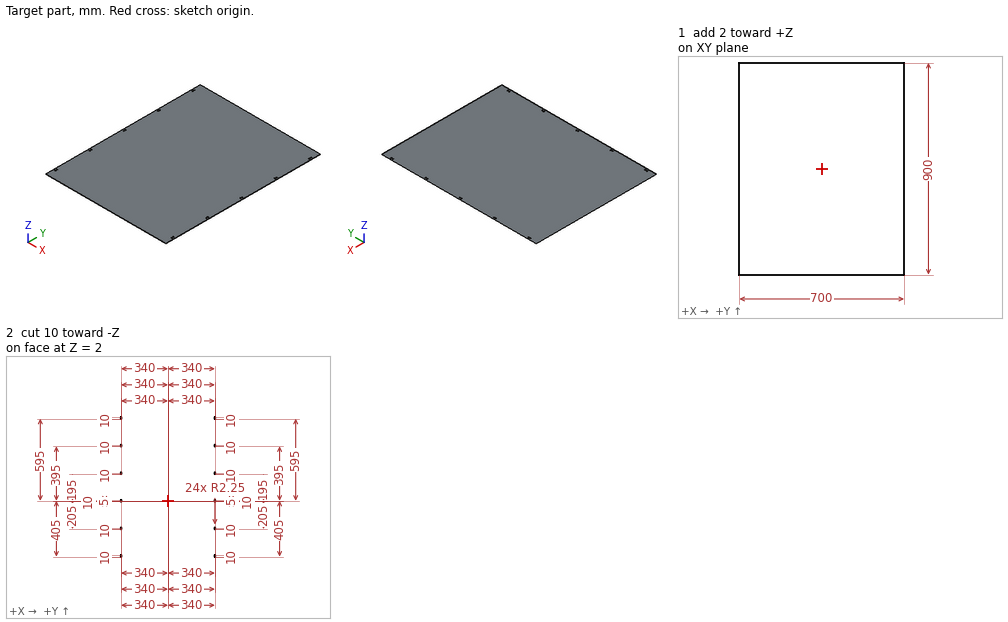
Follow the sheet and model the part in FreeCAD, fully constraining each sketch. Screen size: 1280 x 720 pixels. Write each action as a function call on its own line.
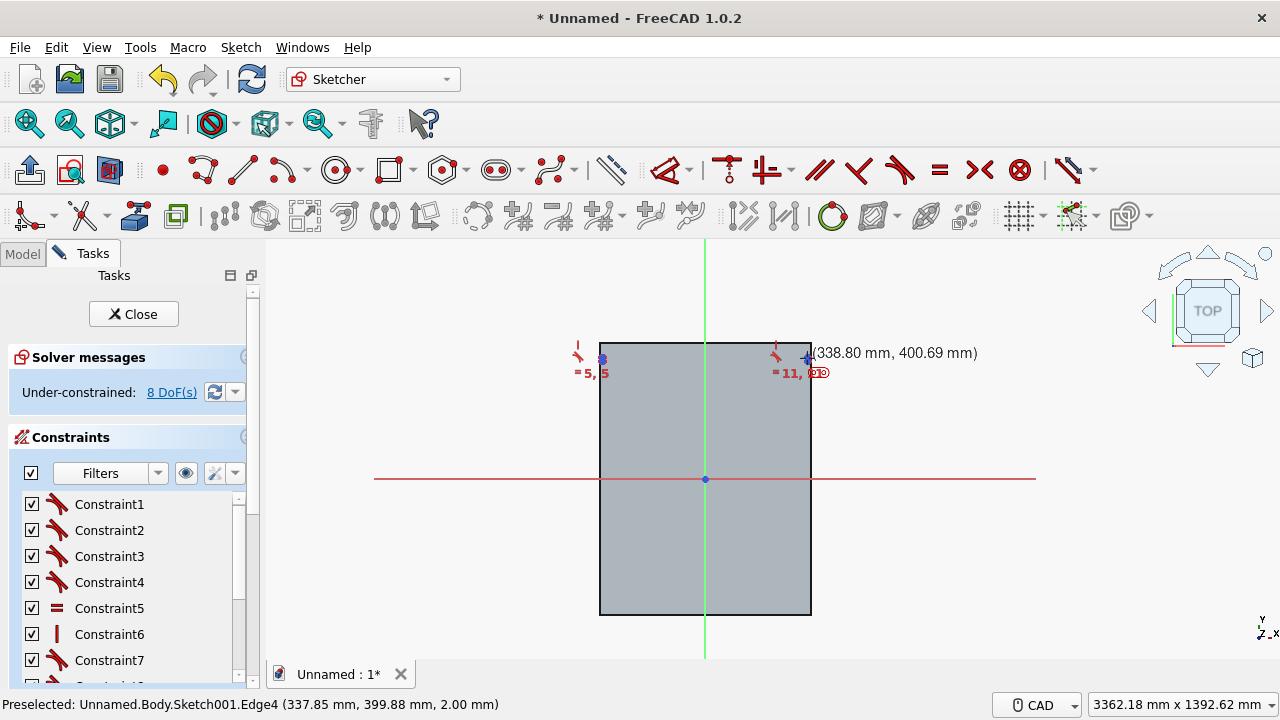
scroll(603, 420, up, 18)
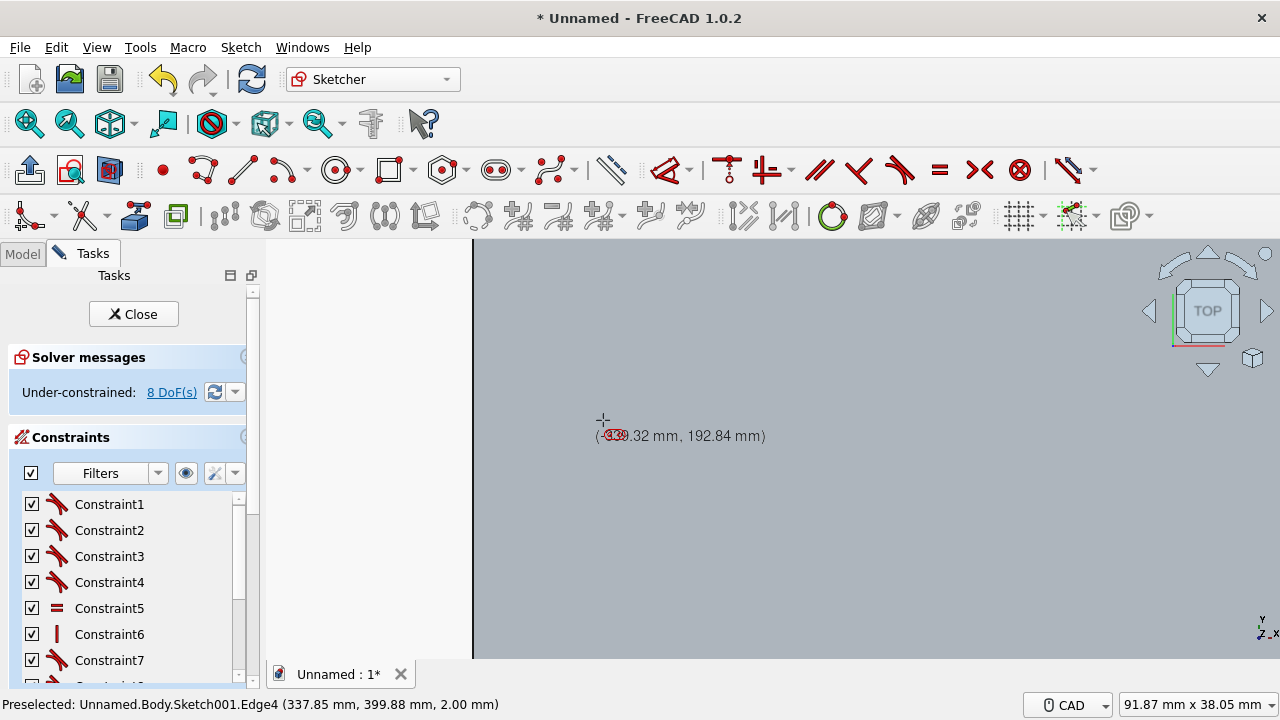
scroll(602, 420, down, 18)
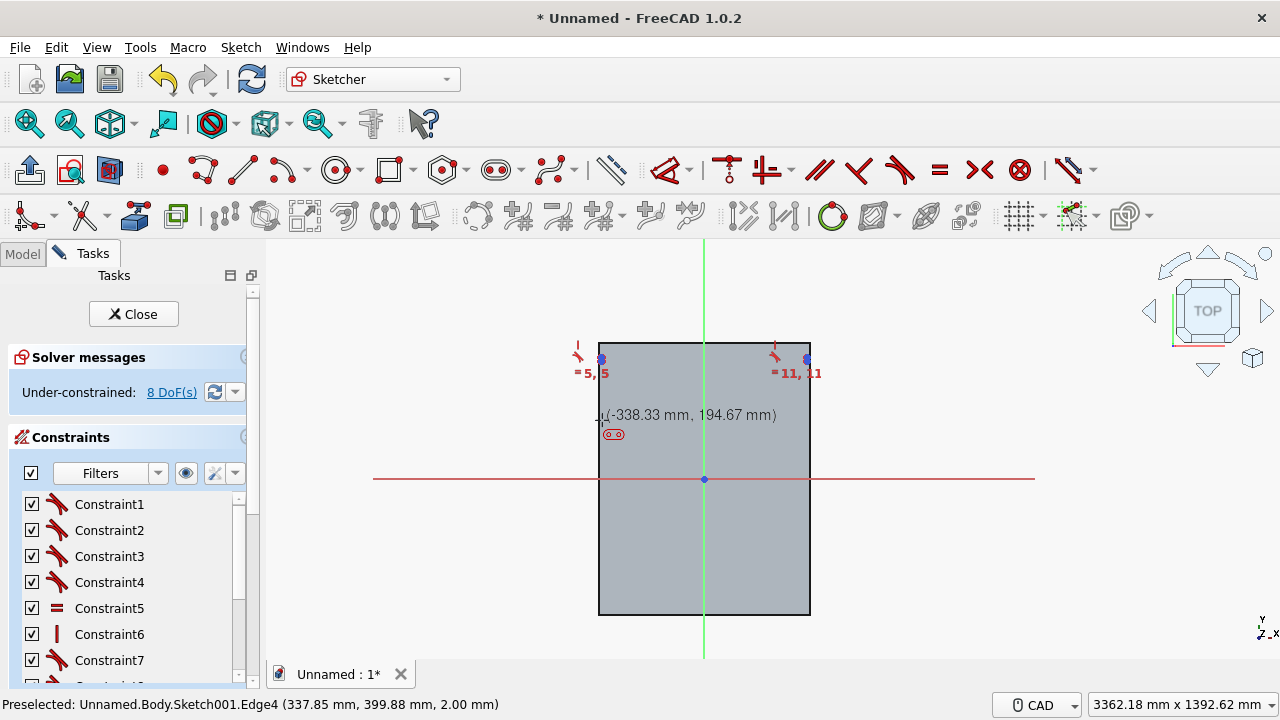
click(602, 420)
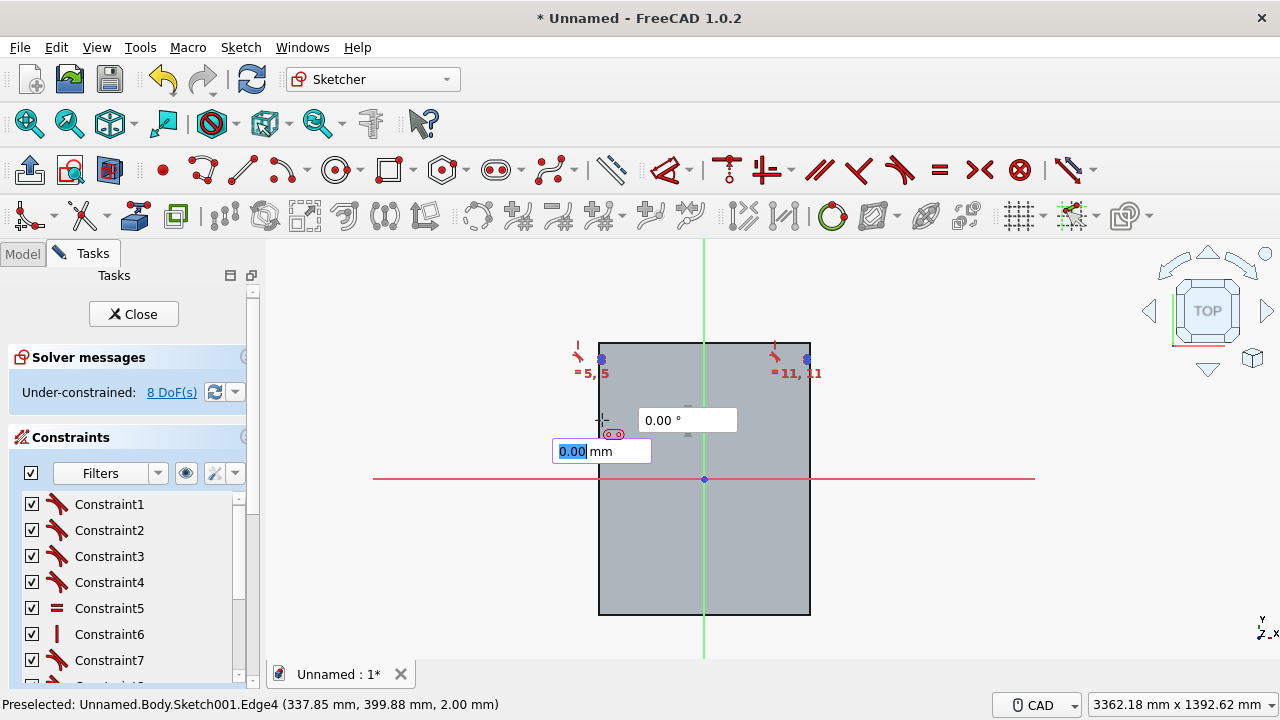
scroll(602, 417, up, 9)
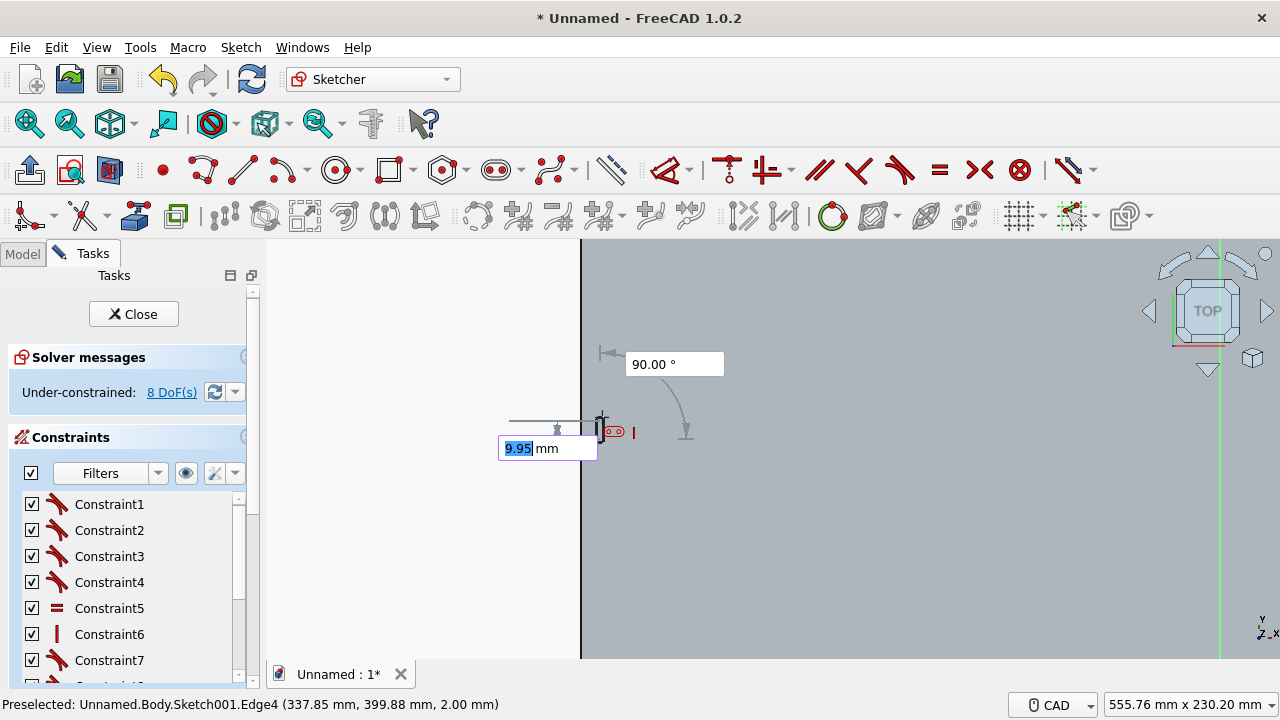
click(600, 417)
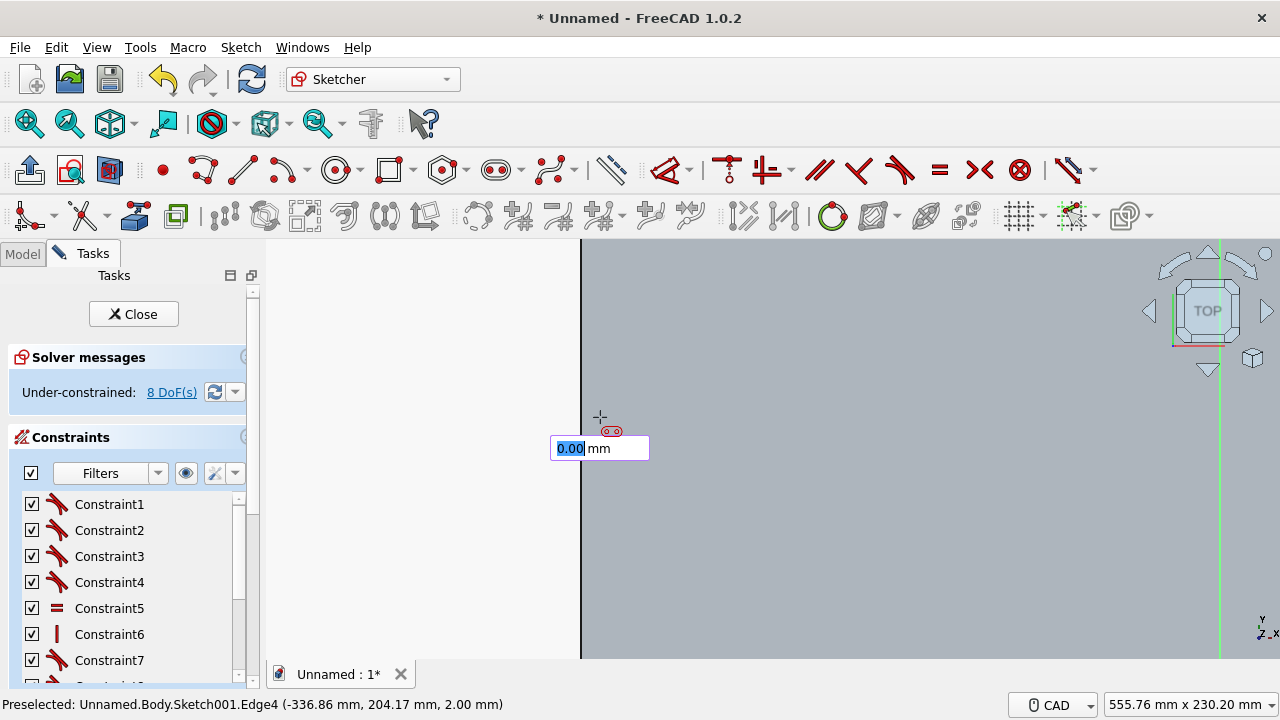
scroll(595, 426, up, 7)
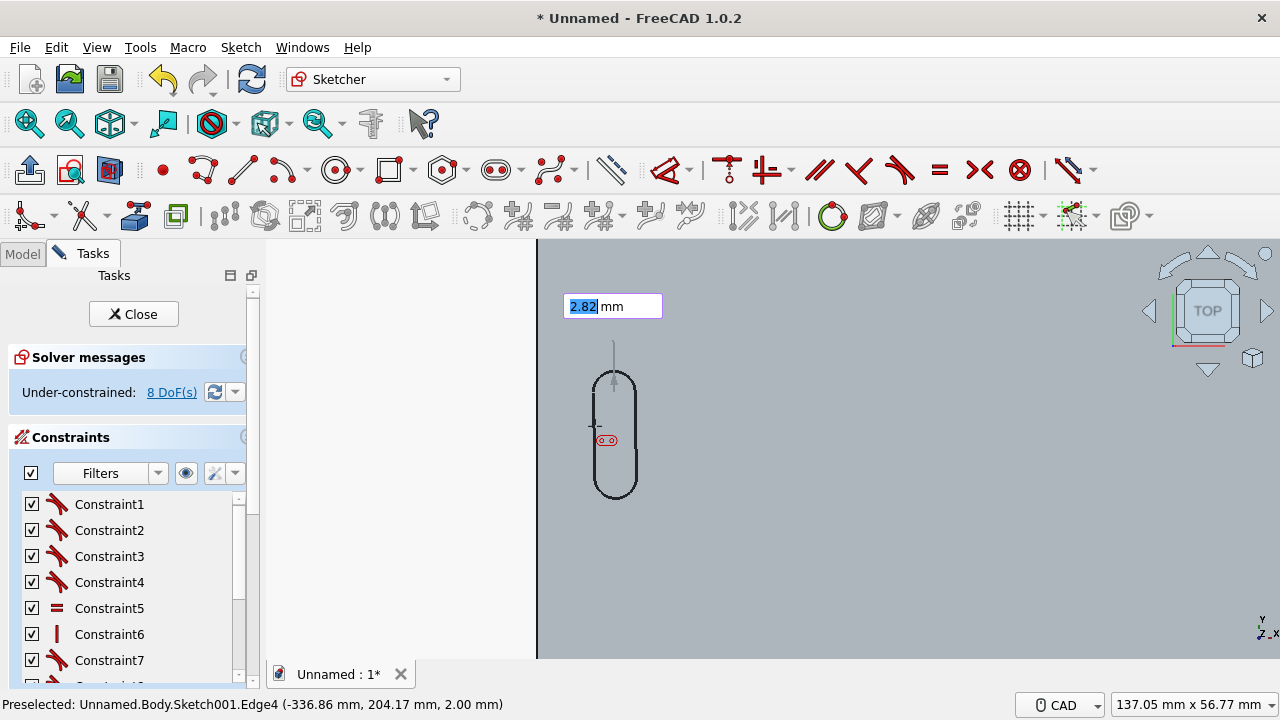
click(595, 425)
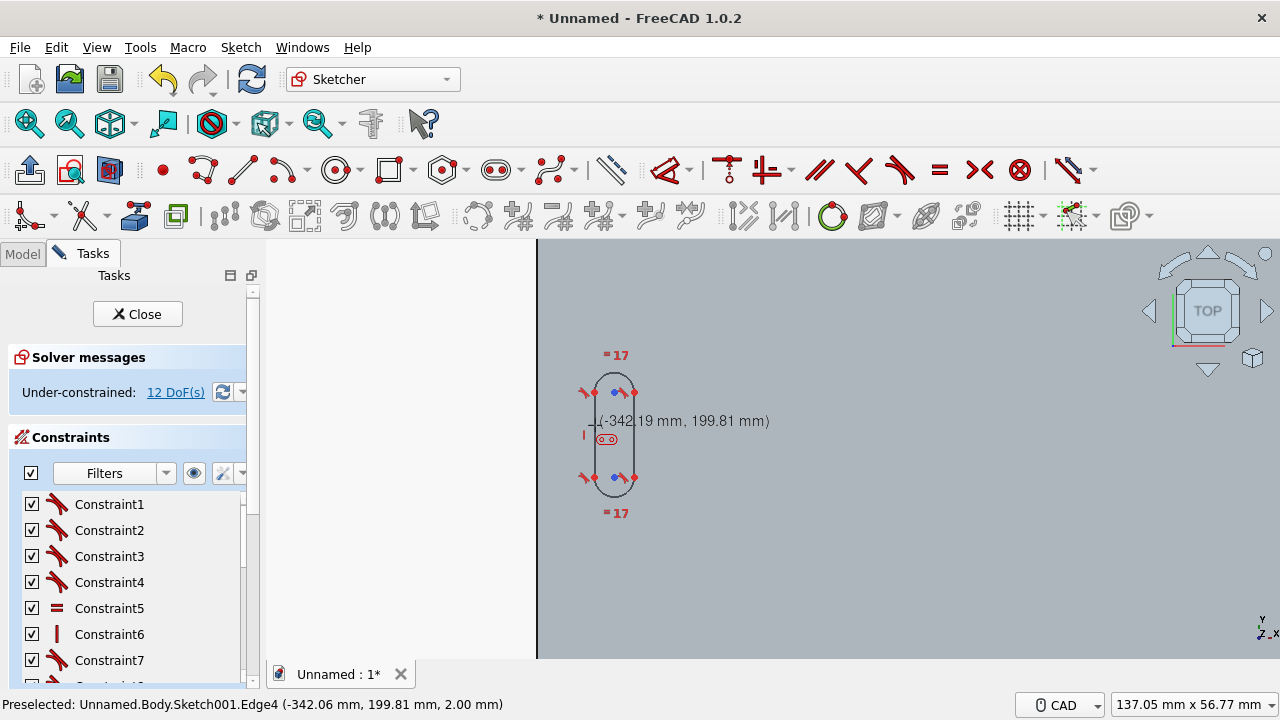
scroll(602, 419, down, 16)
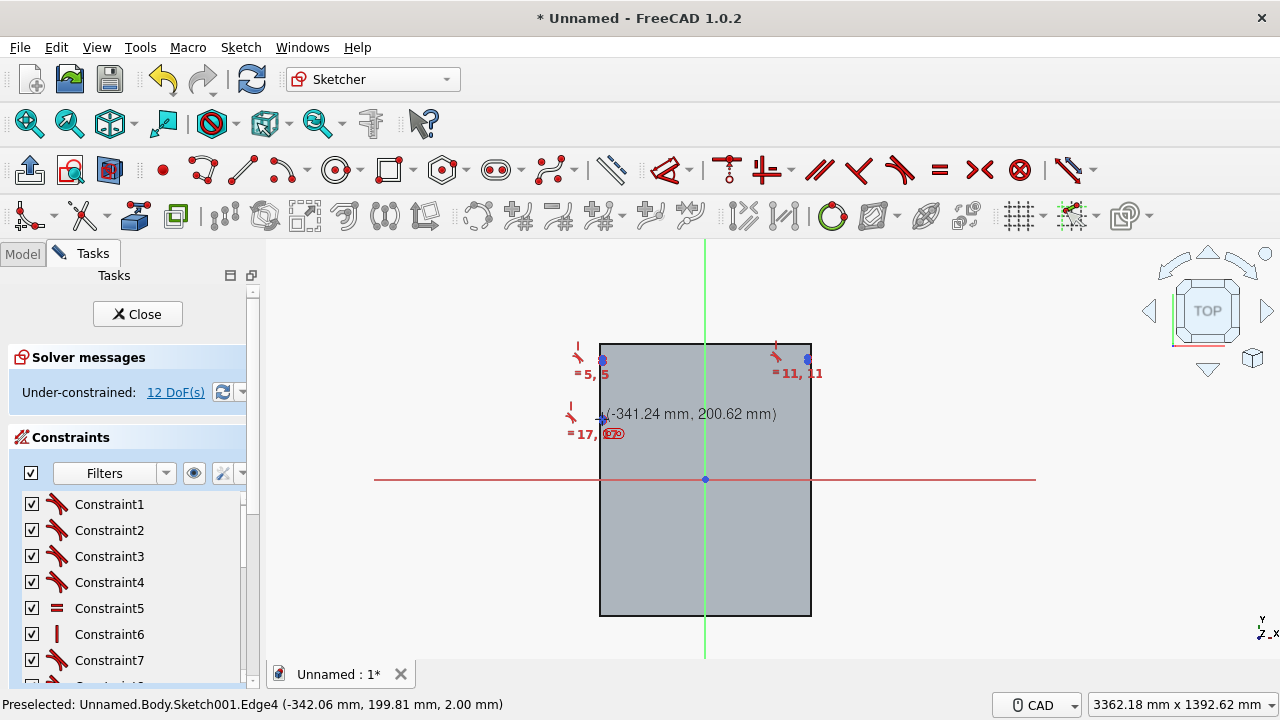
scroll(603, 481, up, 18)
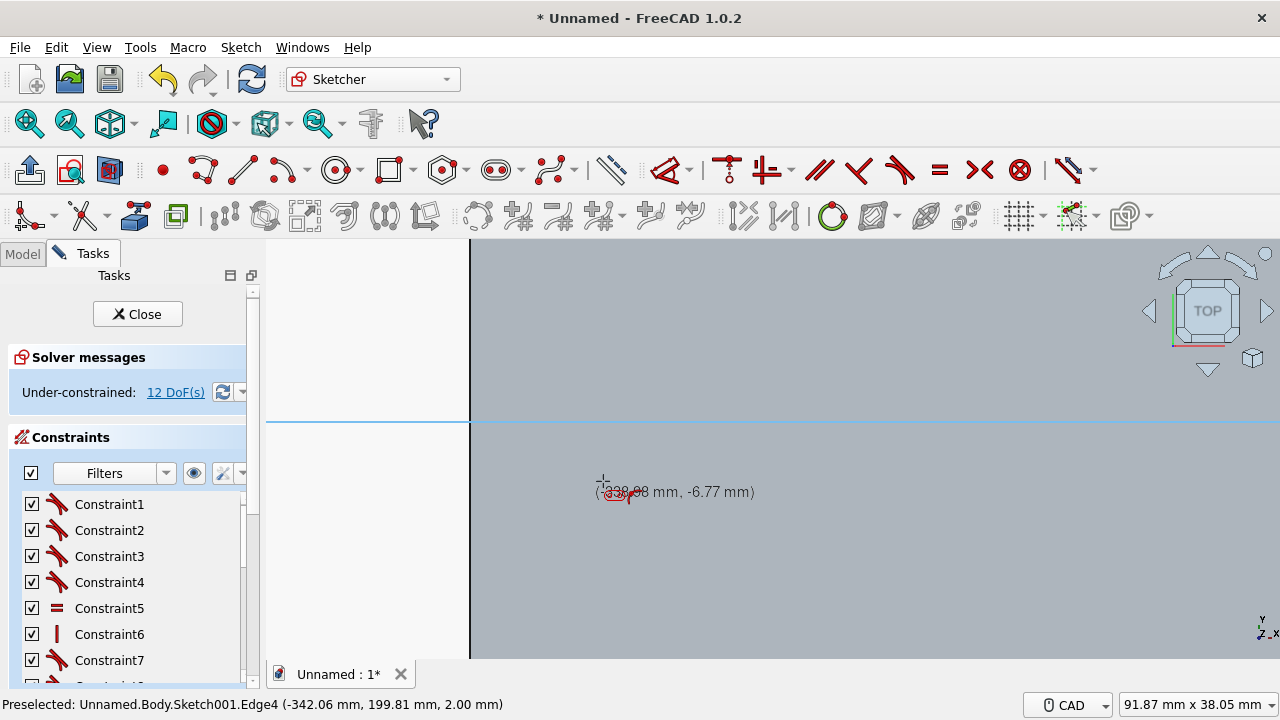
scroll(603, 481, down, 18)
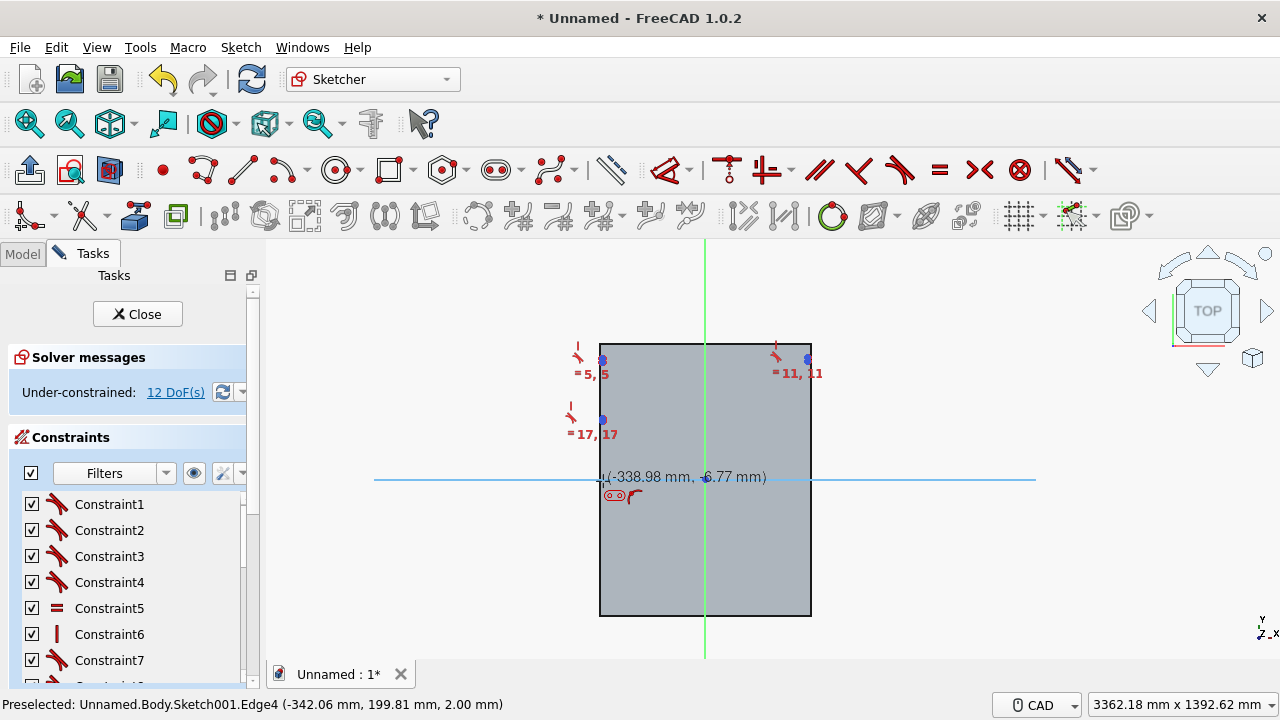
scroll(603, 481, up, 12)